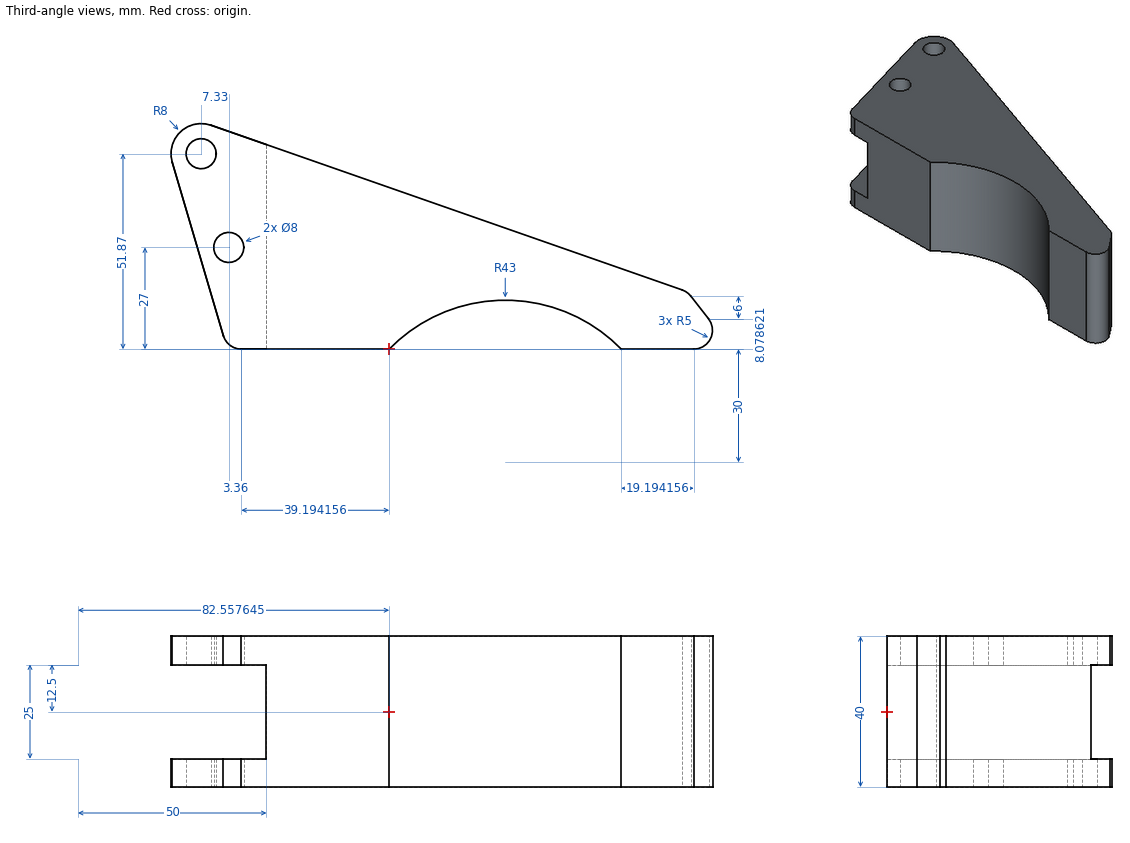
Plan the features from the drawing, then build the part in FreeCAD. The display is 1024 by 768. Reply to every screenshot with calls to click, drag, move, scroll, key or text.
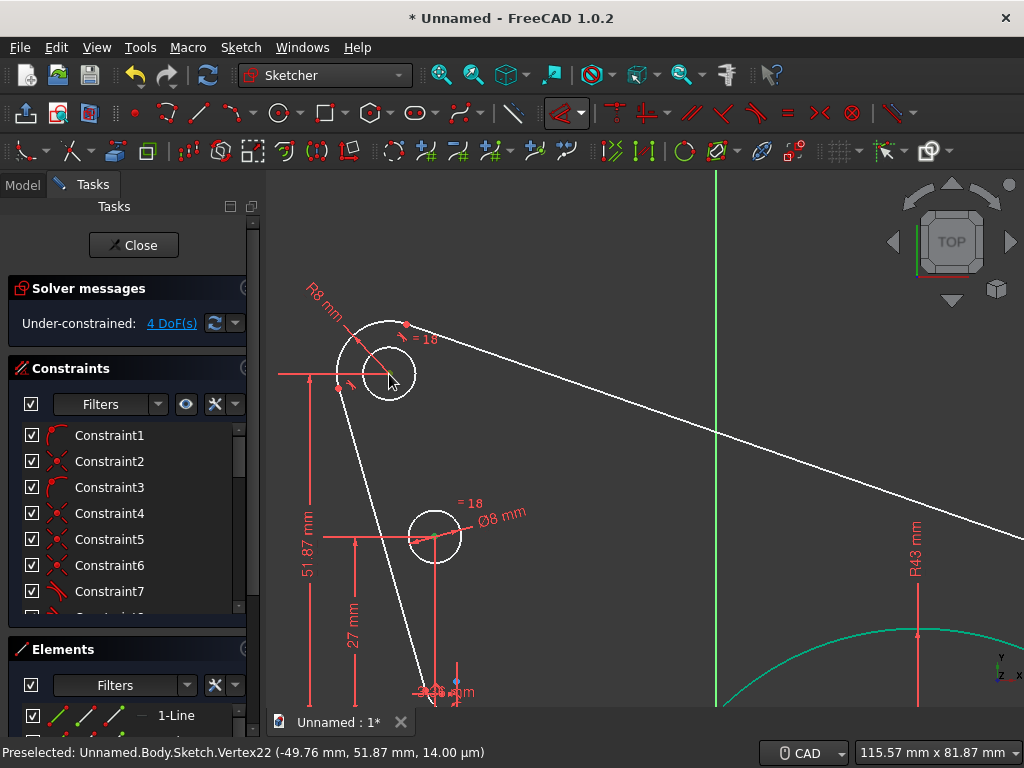
key(l)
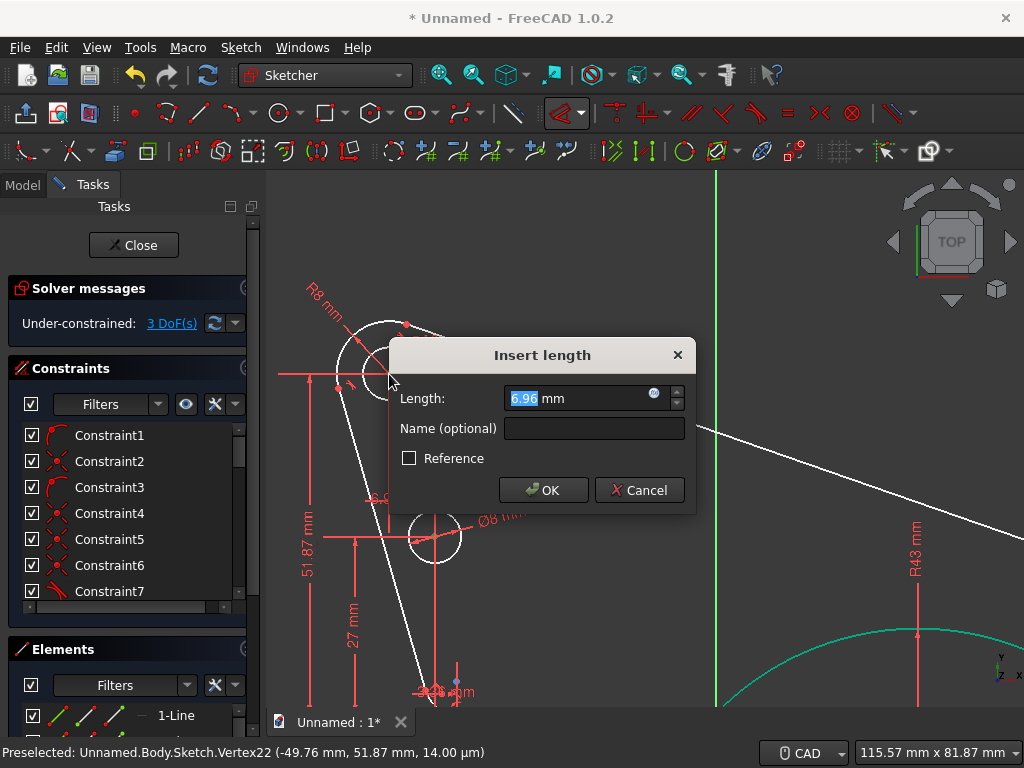
text(7.33)
key(Return)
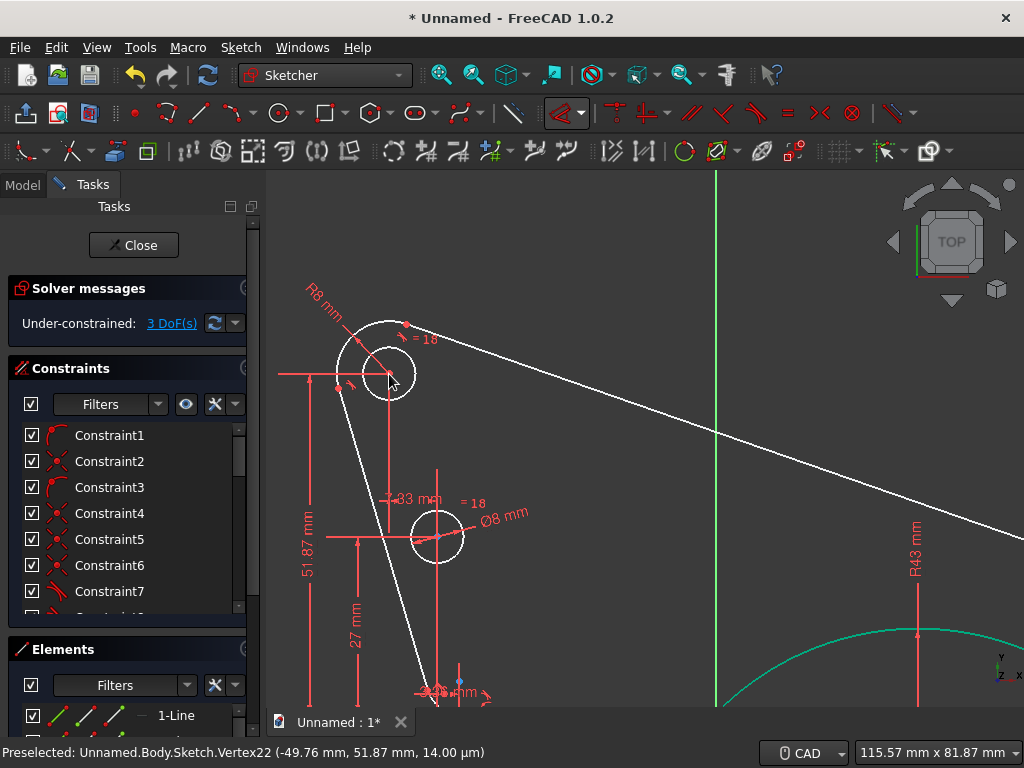
scroll(389, 373, down, 4)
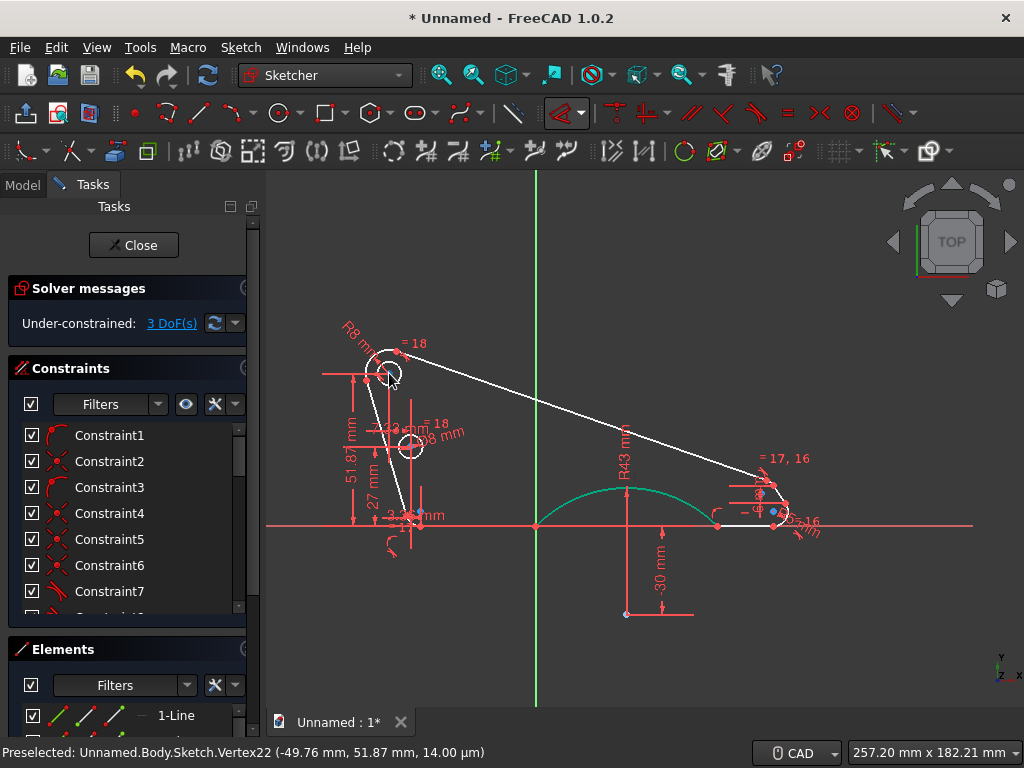
click(455, 526)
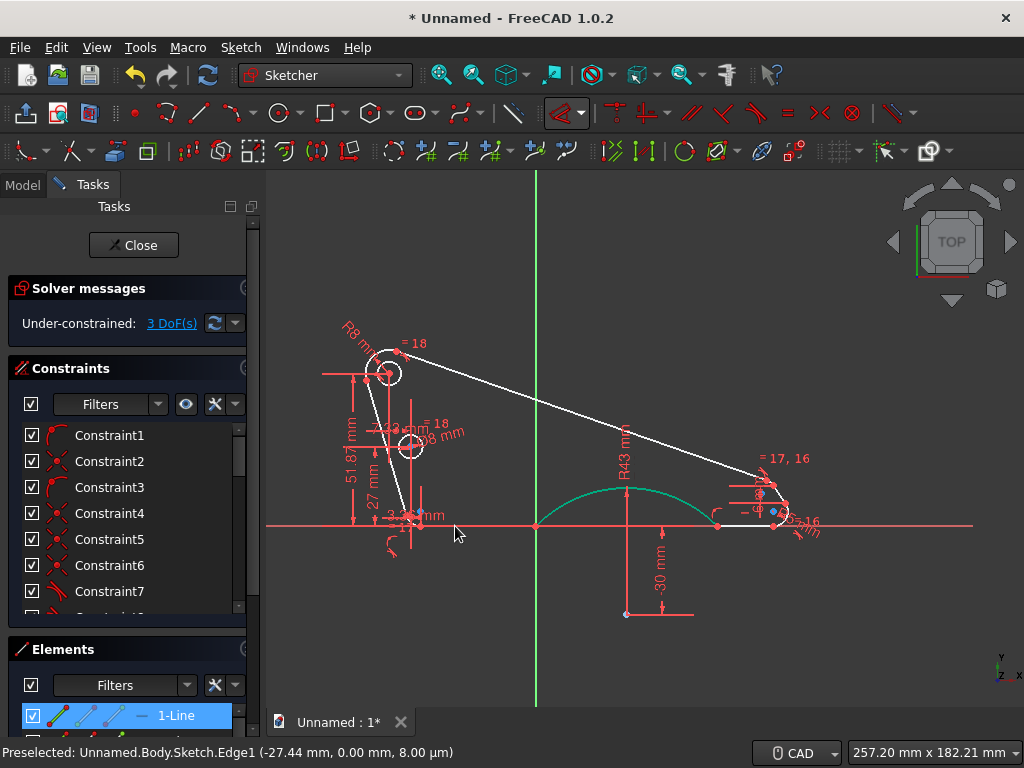
click(584, 114)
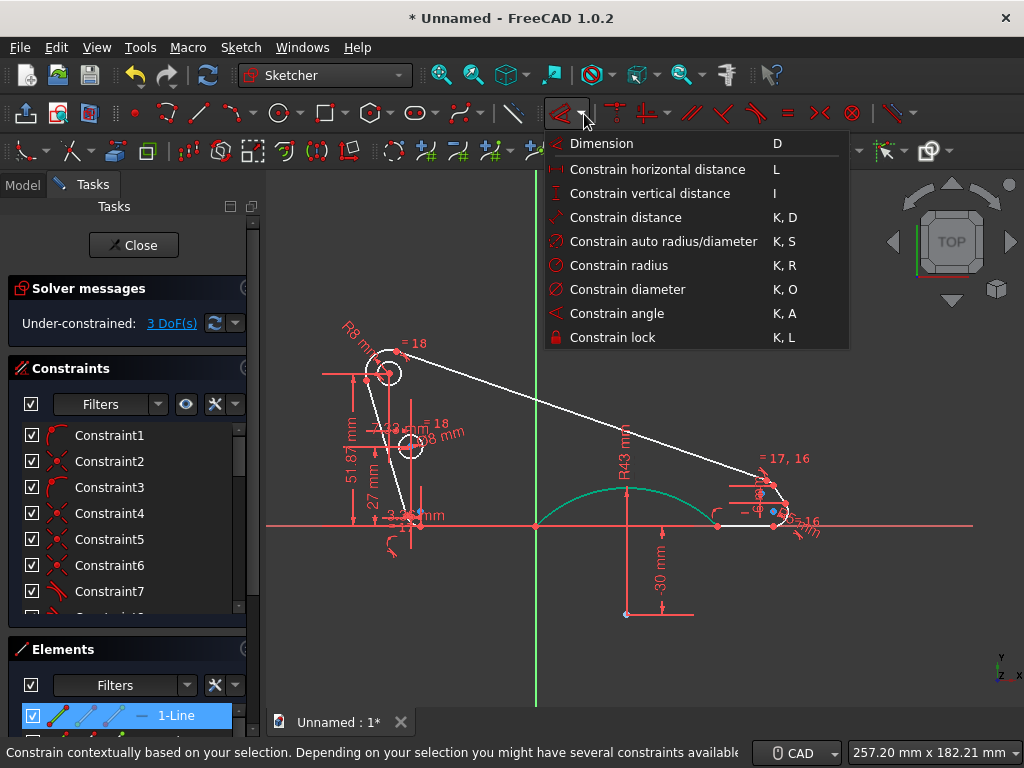
click(697, 169)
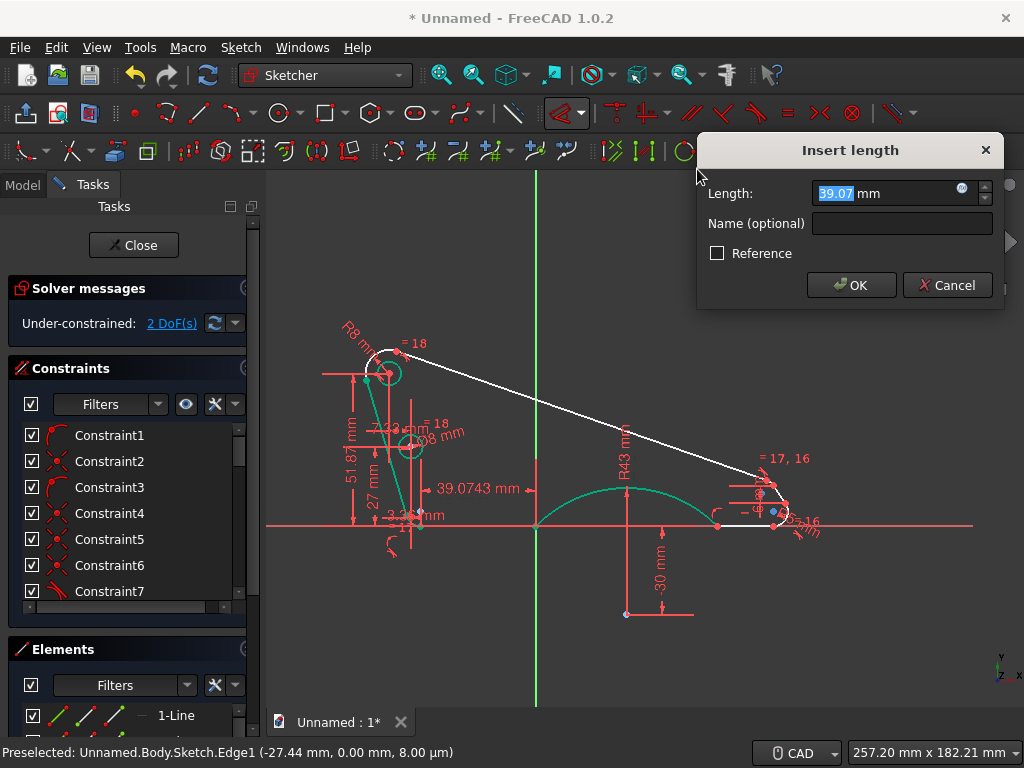
text(39.194156)
key(Return)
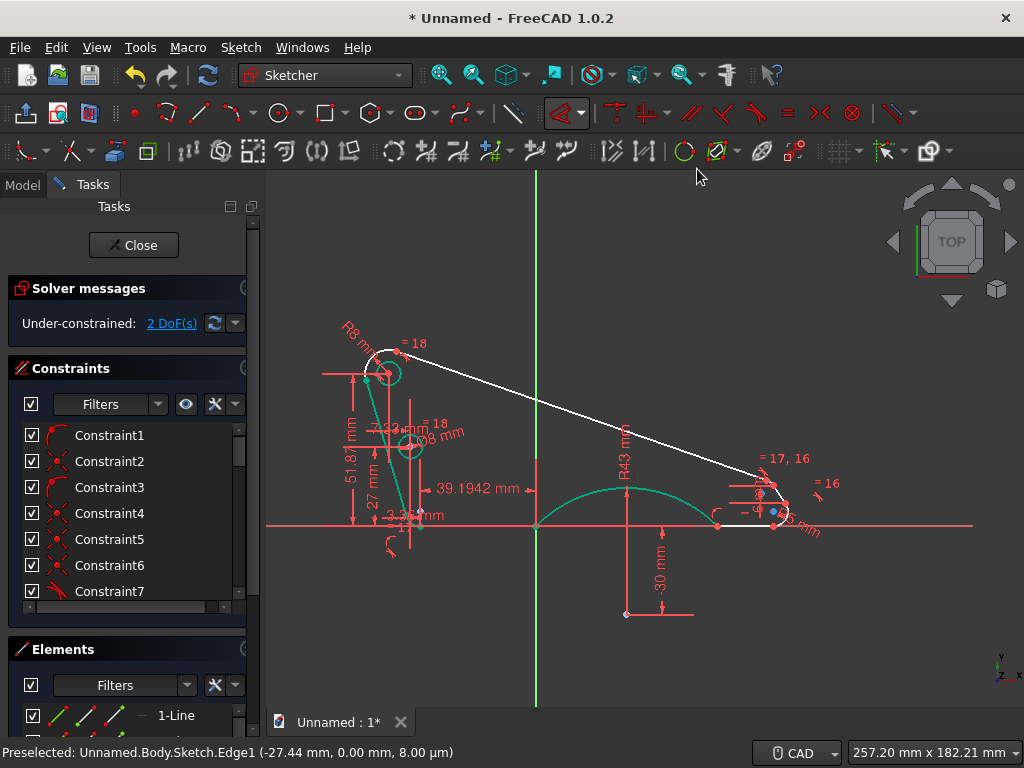
click(734, 526)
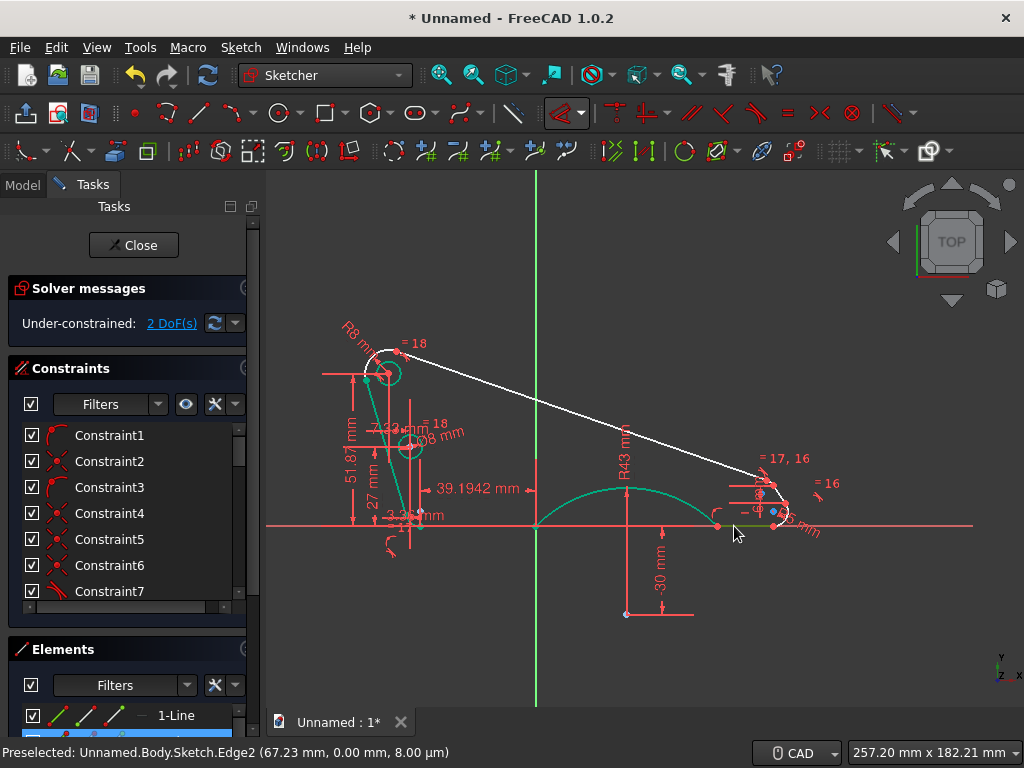
click(584, 114)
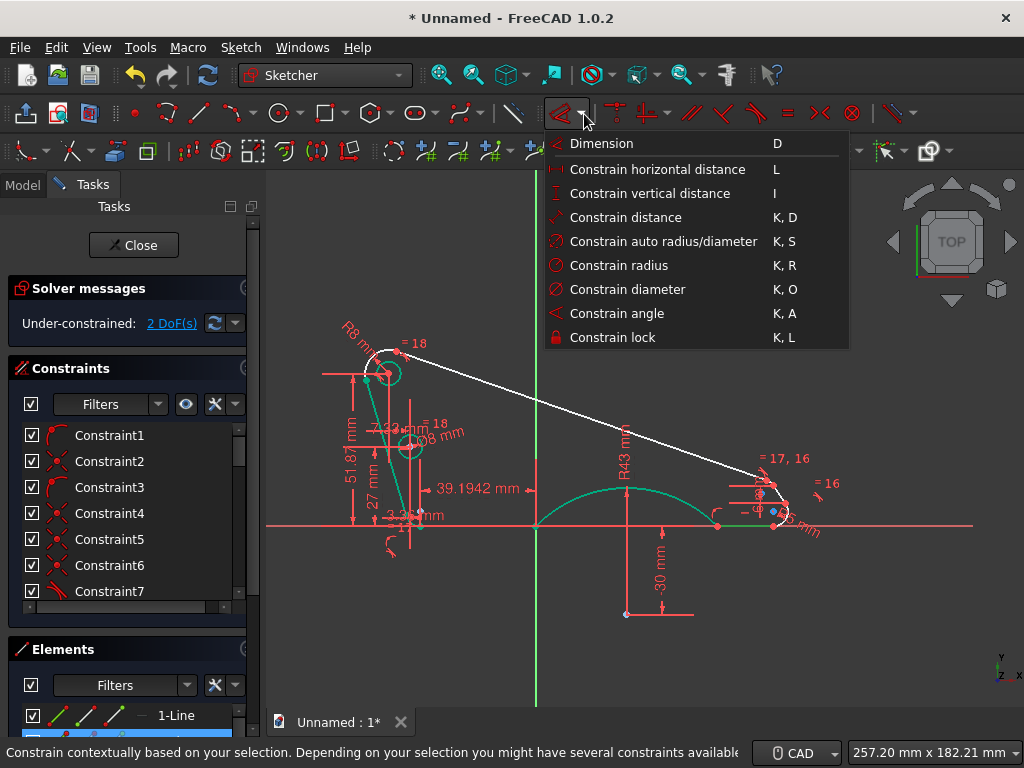
click(697, 169)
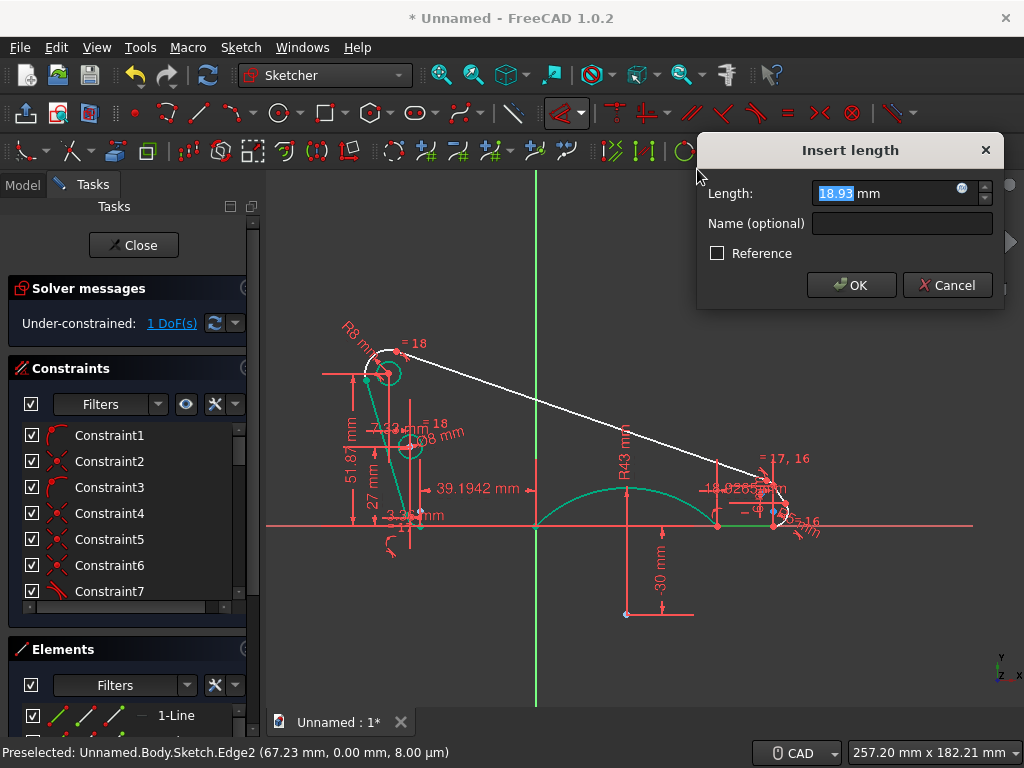
text(19.194156)
key(Return)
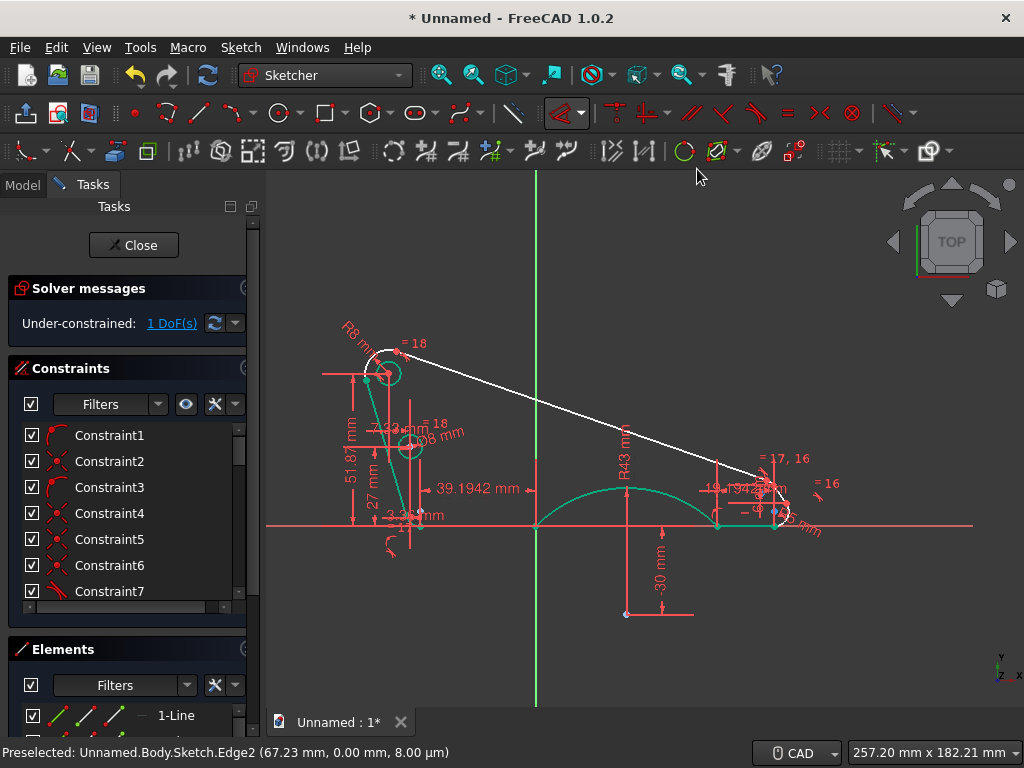
scroll(786, 503, up, 3)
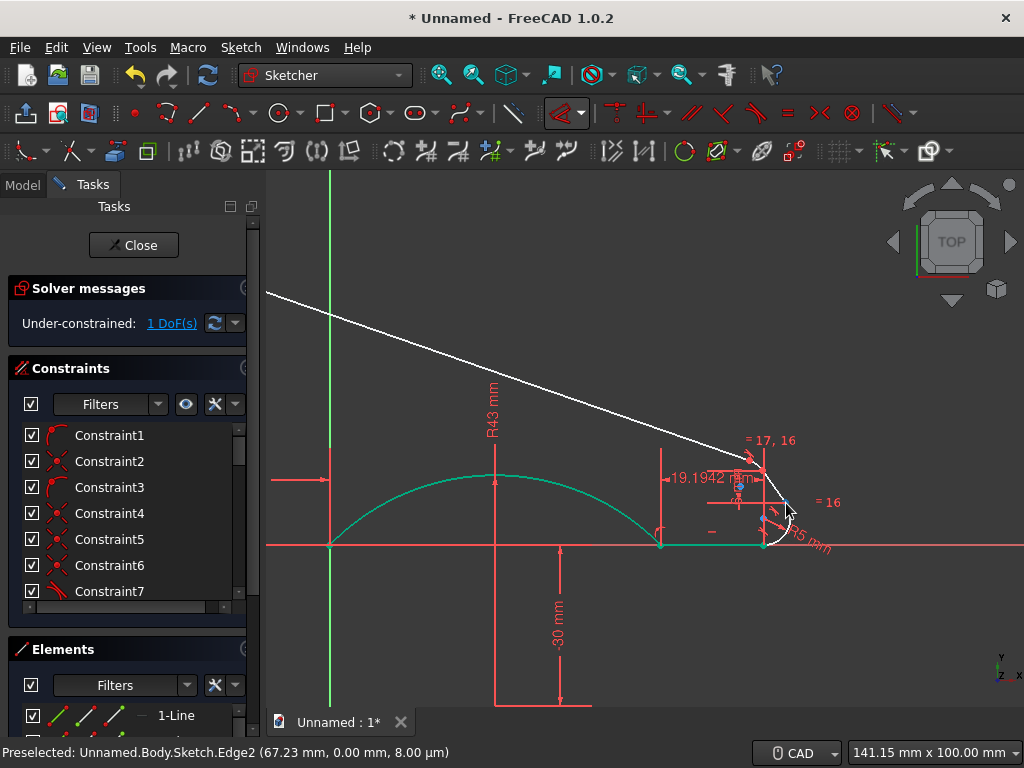
click(786, 503)